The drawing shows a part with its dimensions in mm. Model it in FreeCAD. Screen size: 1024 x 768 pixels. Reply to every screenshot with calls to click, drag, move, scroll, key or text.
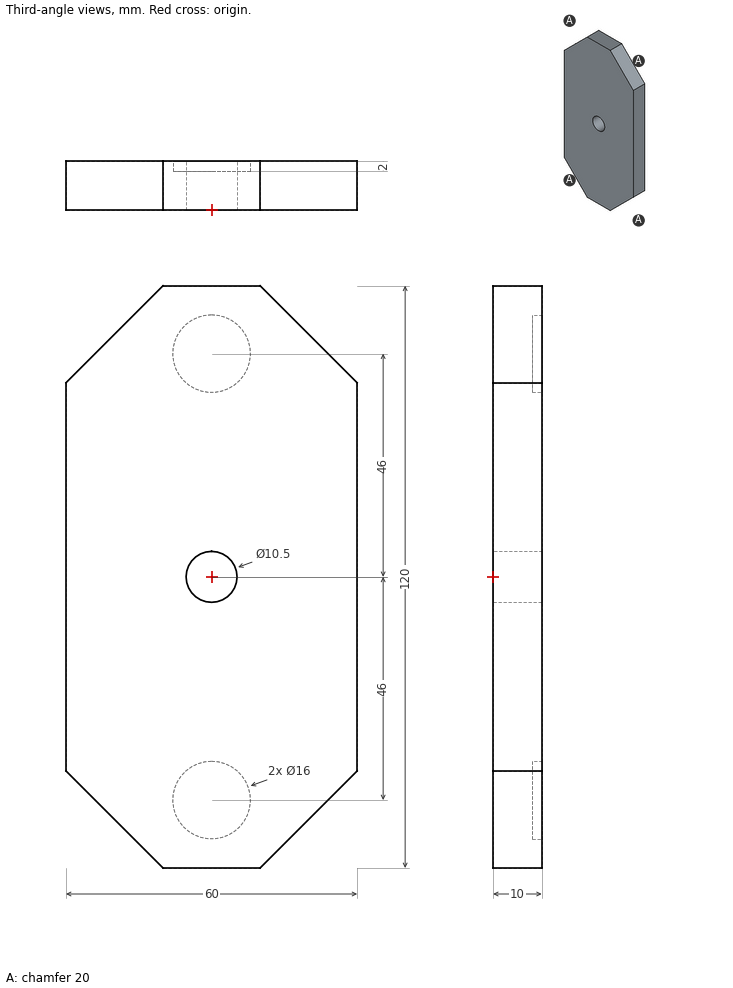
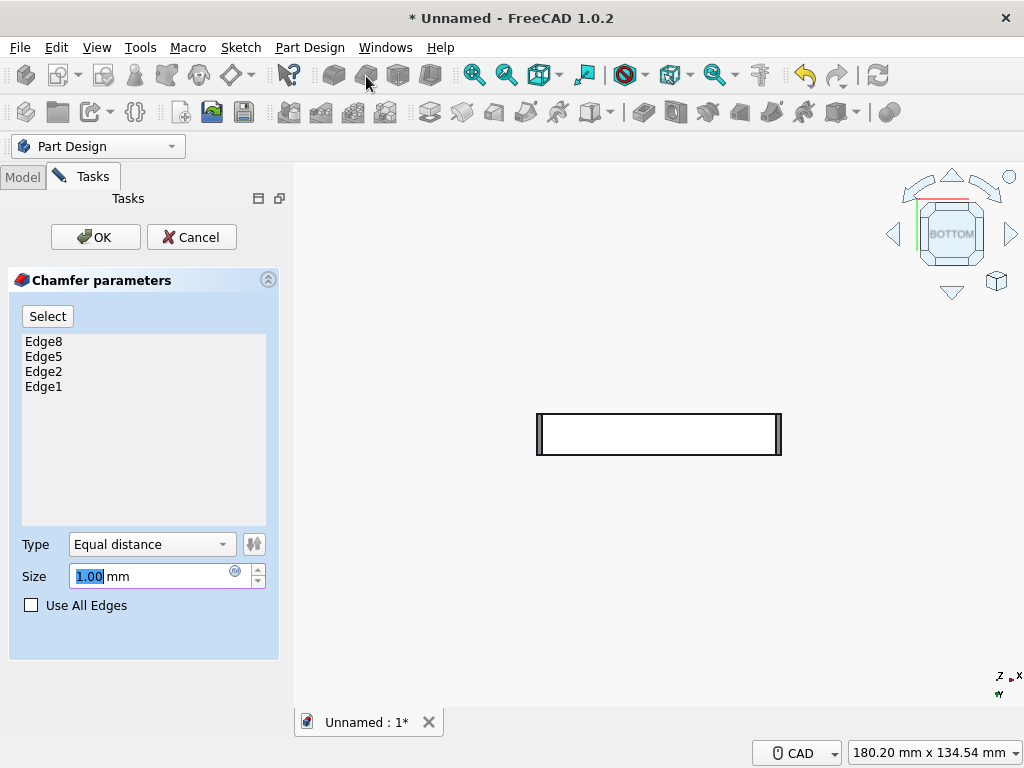
text(20)
key(Tab)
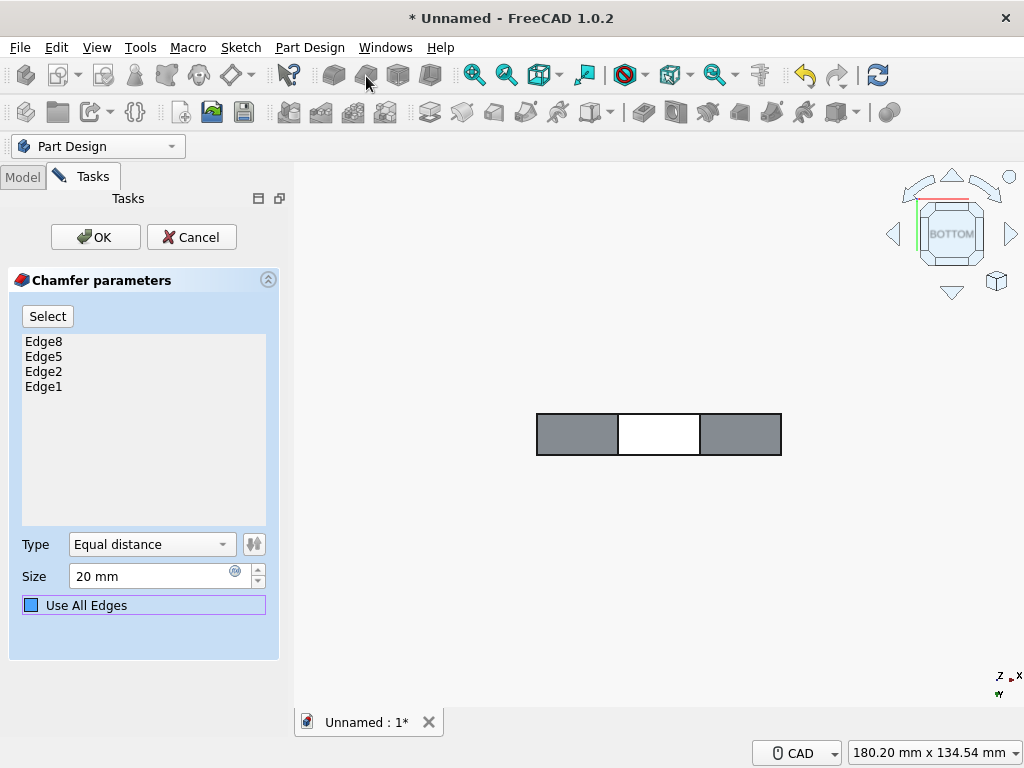
click(96, 237)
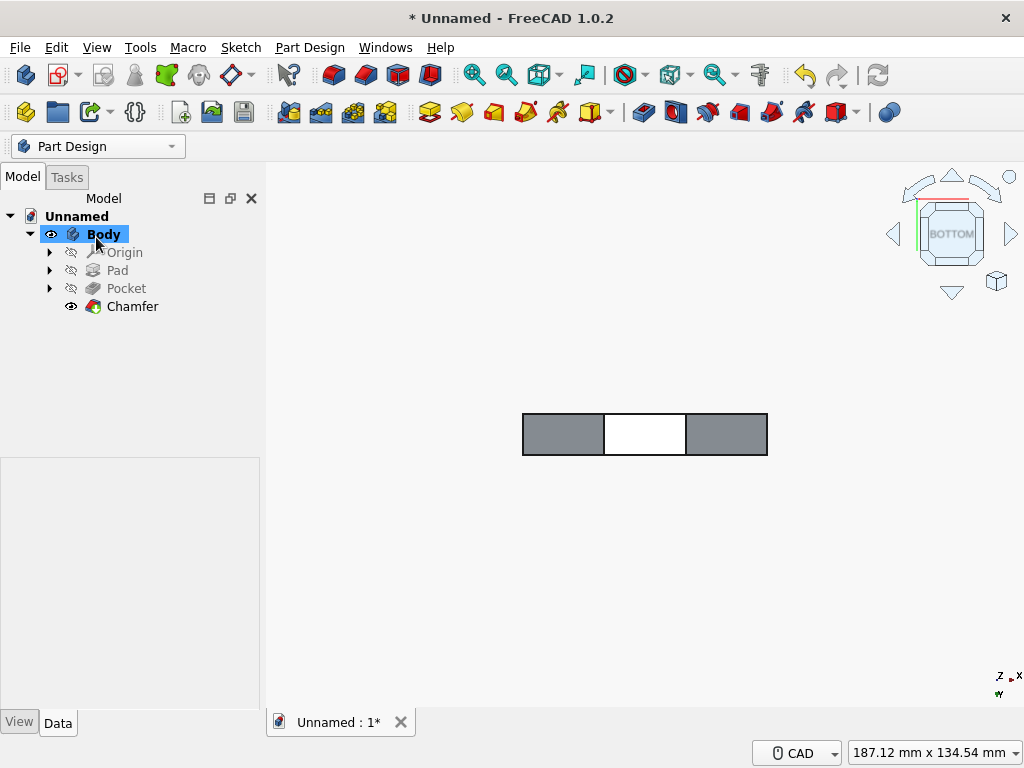
click(476, 76)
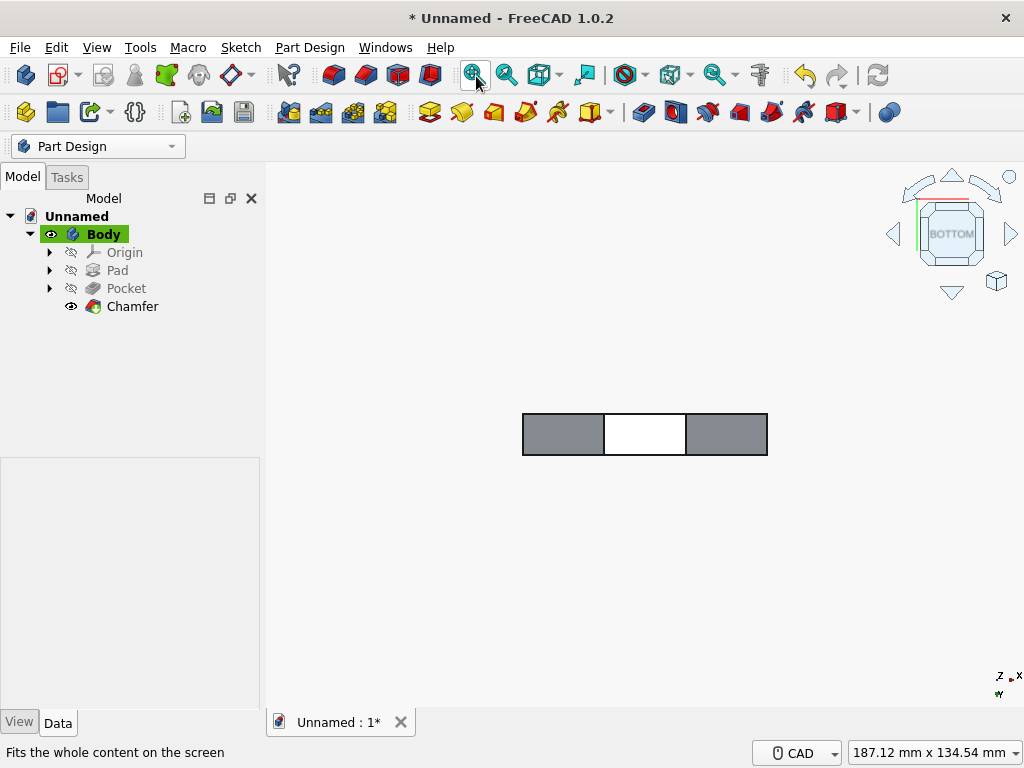
key(4)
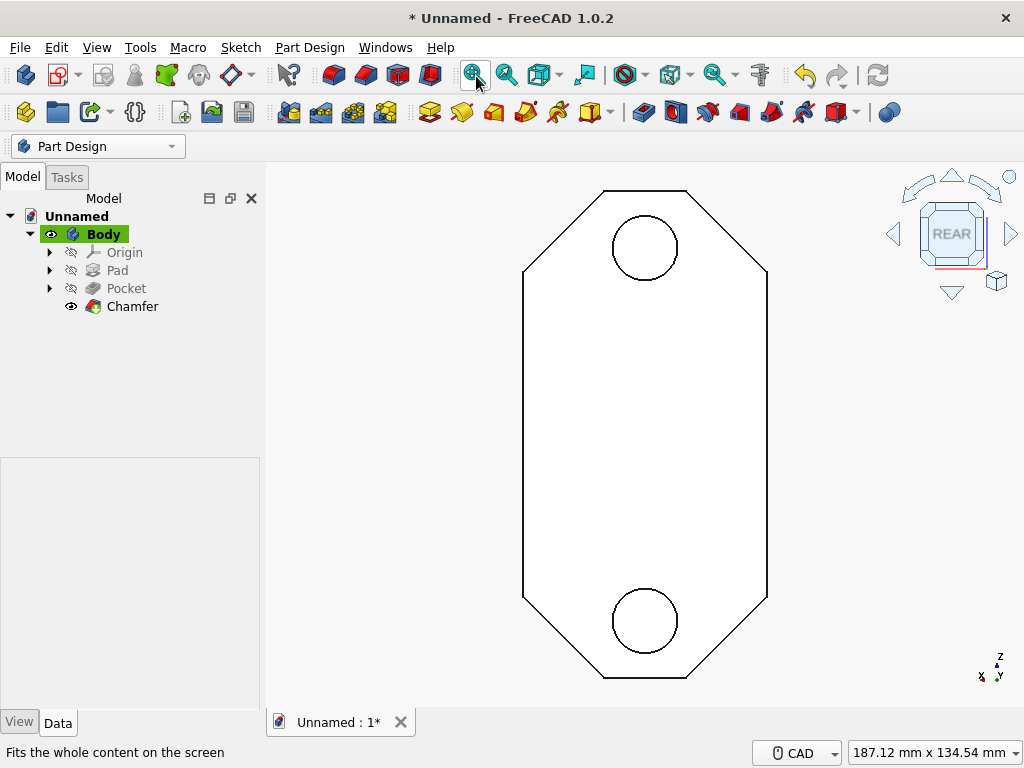
click(645, 433)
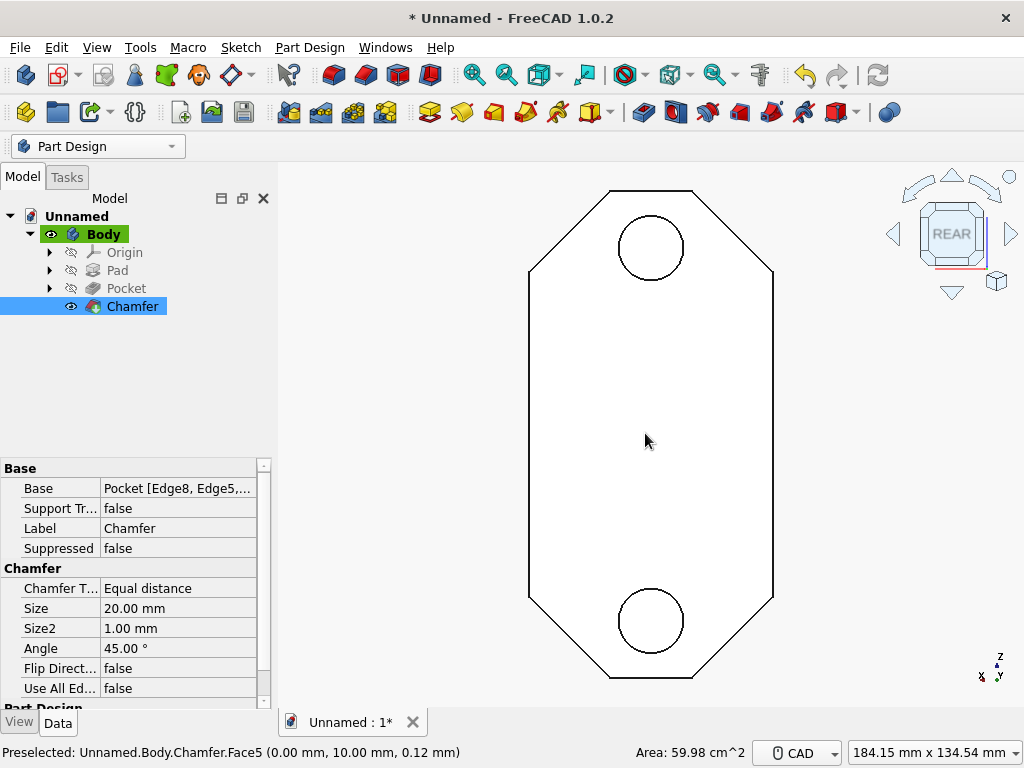
click(58, 76)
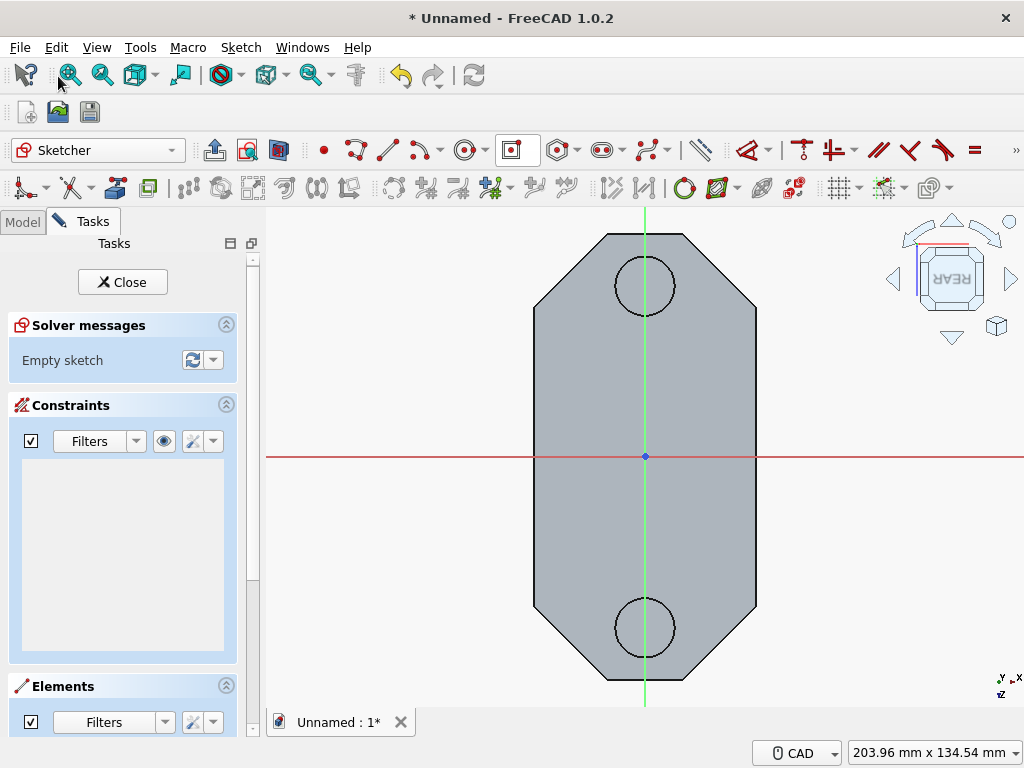
scroll(656, 457, up, 10)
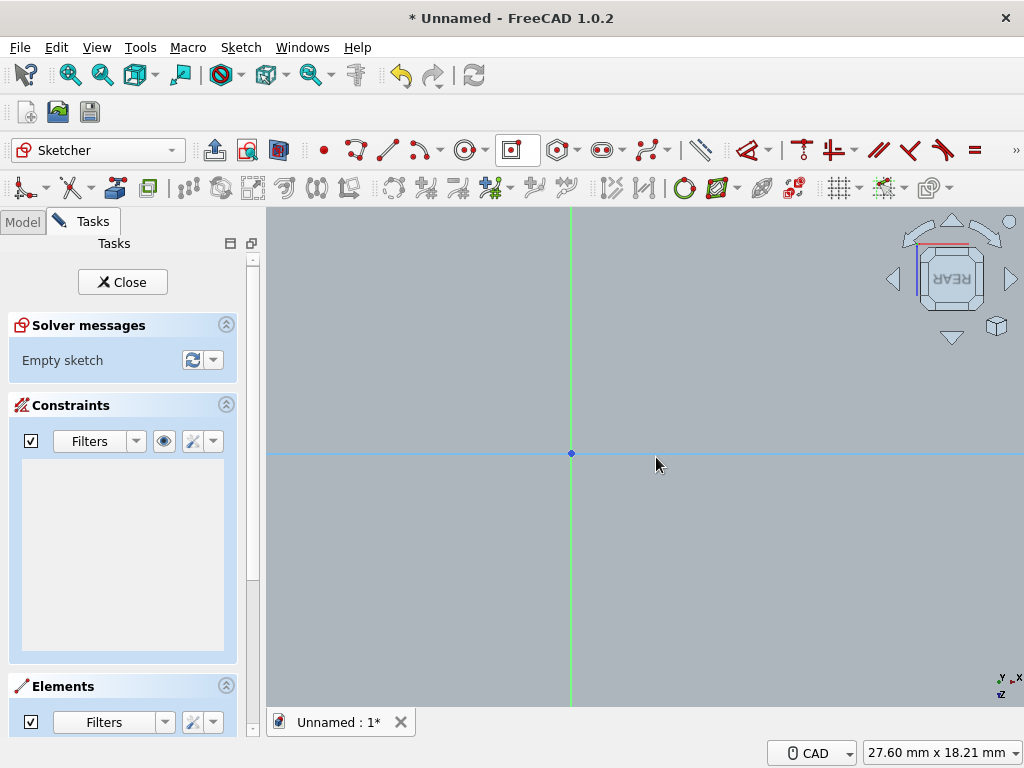
click(466, 150)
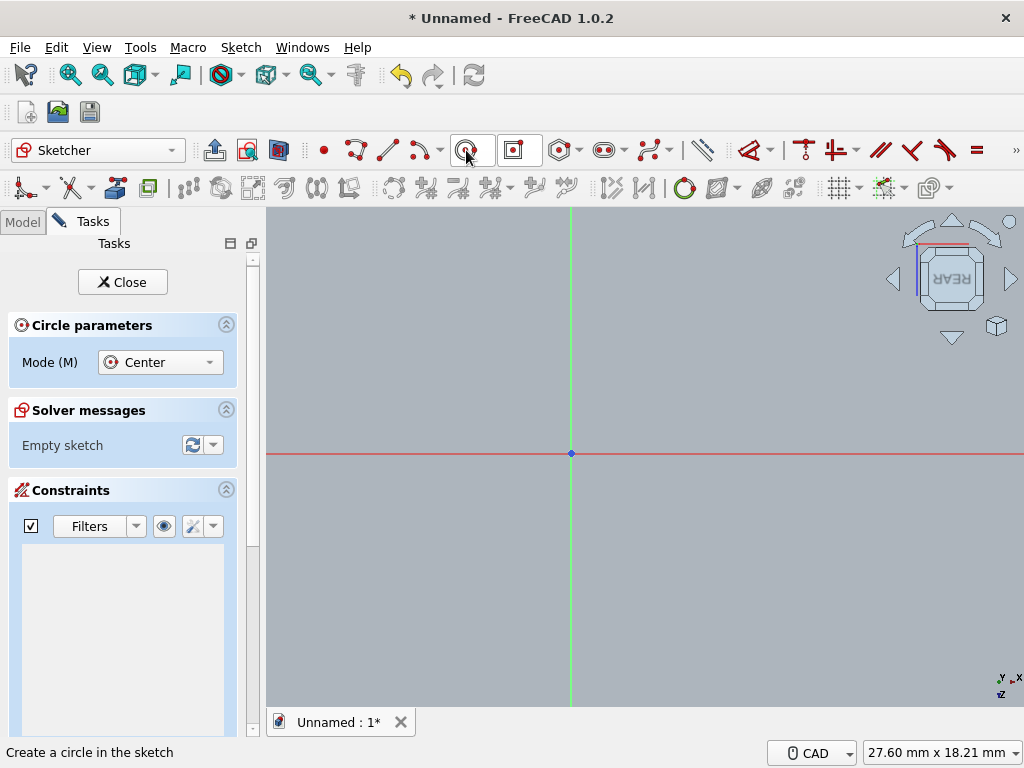
click(571, 454)
click(673, 352)
key(Escape)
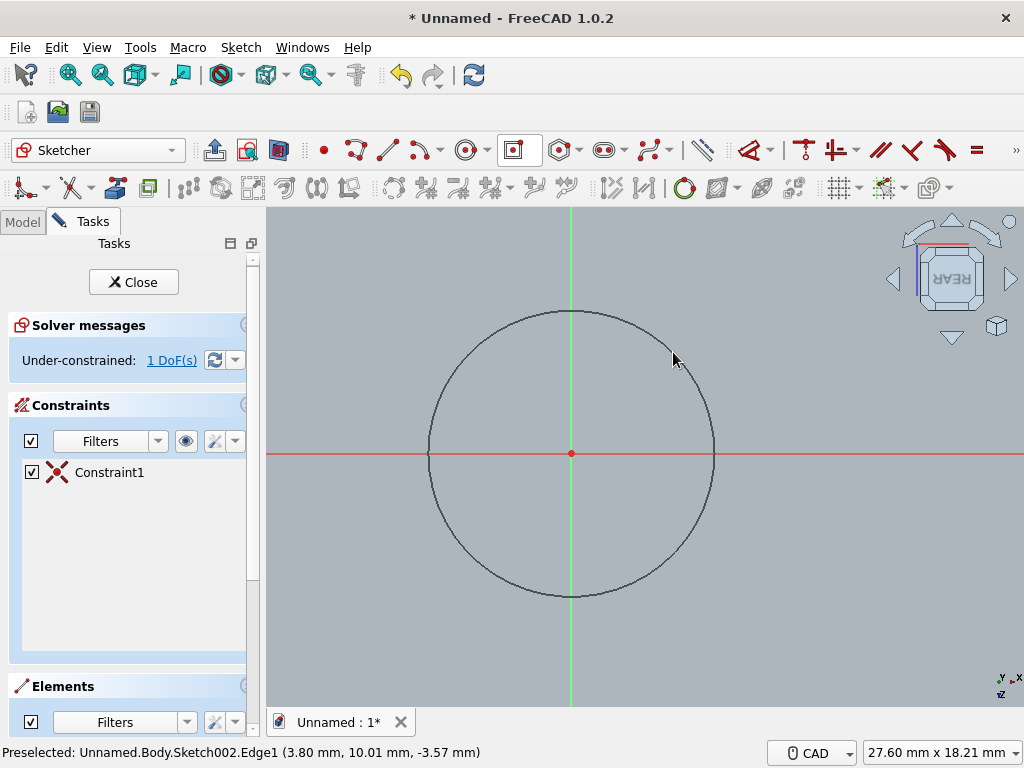
click(750, 150)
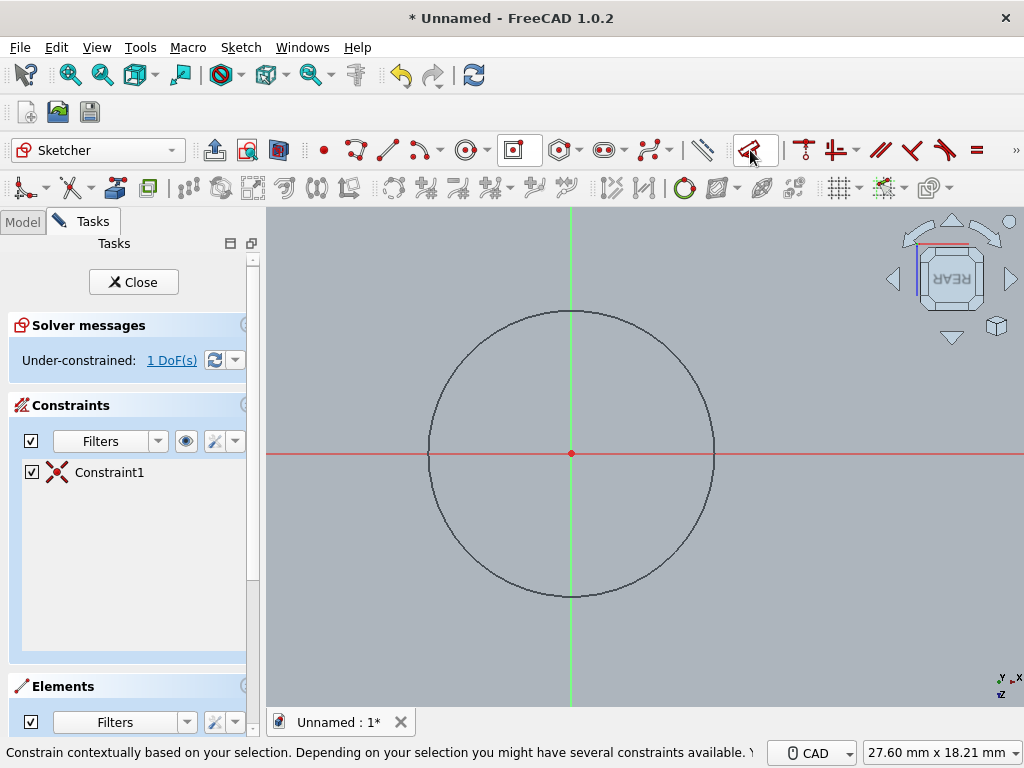
click(672, 352)
click(694, 329)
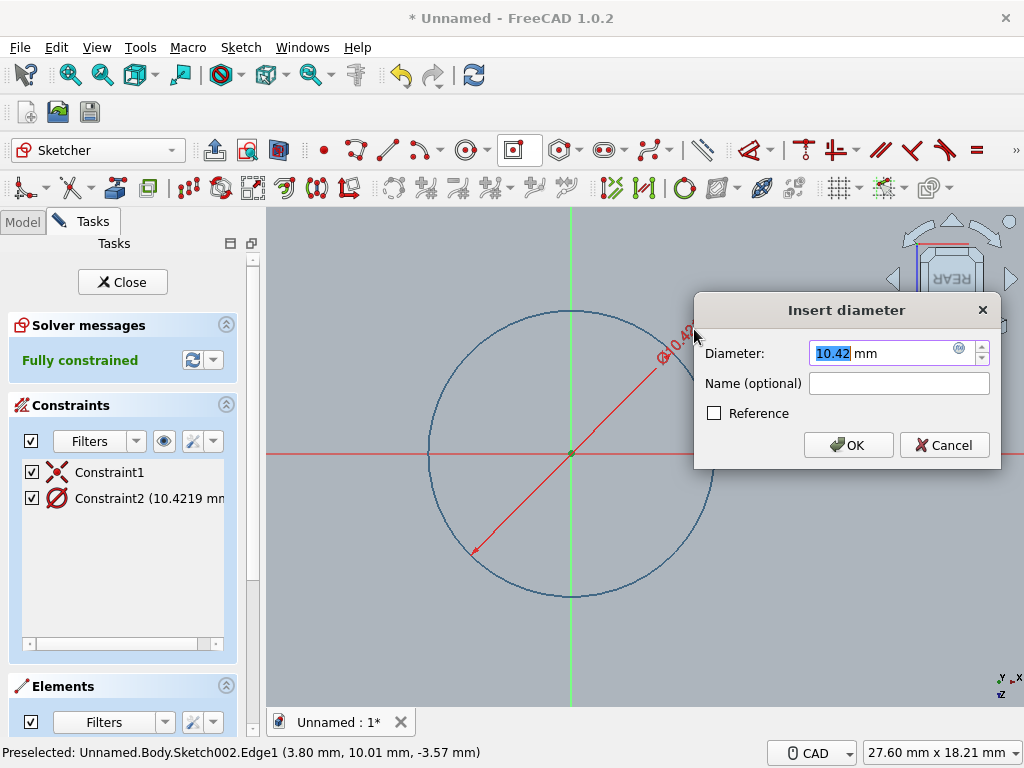
text(10.5)
key(Return)
key(Escape)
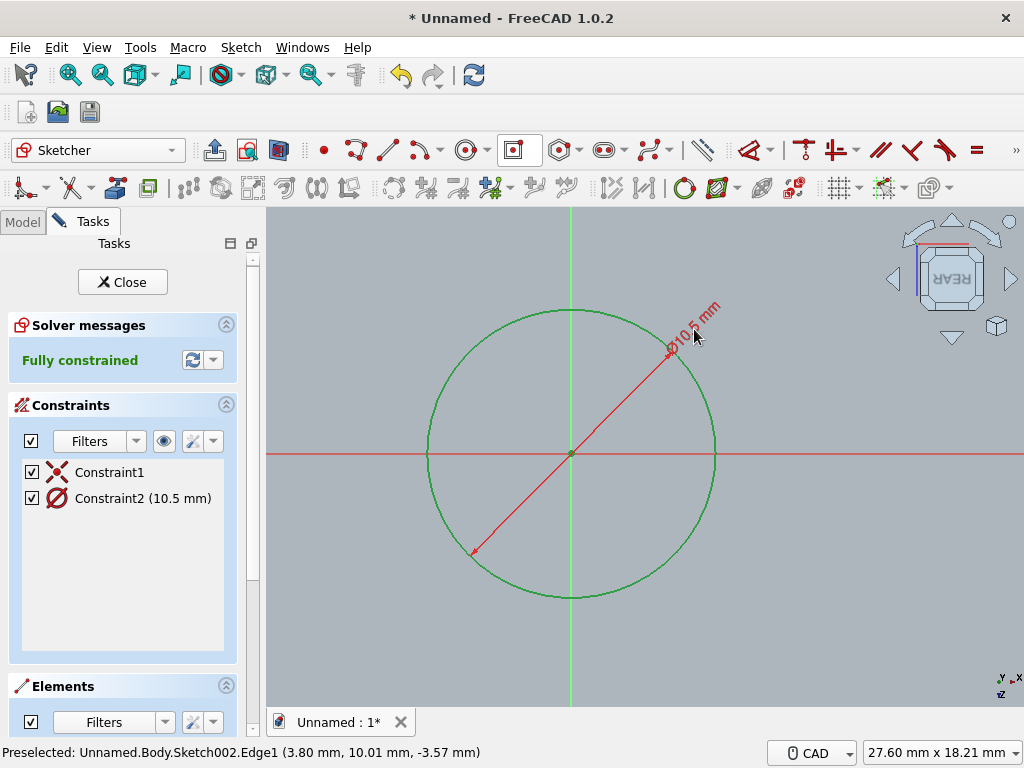
click(123, 282)